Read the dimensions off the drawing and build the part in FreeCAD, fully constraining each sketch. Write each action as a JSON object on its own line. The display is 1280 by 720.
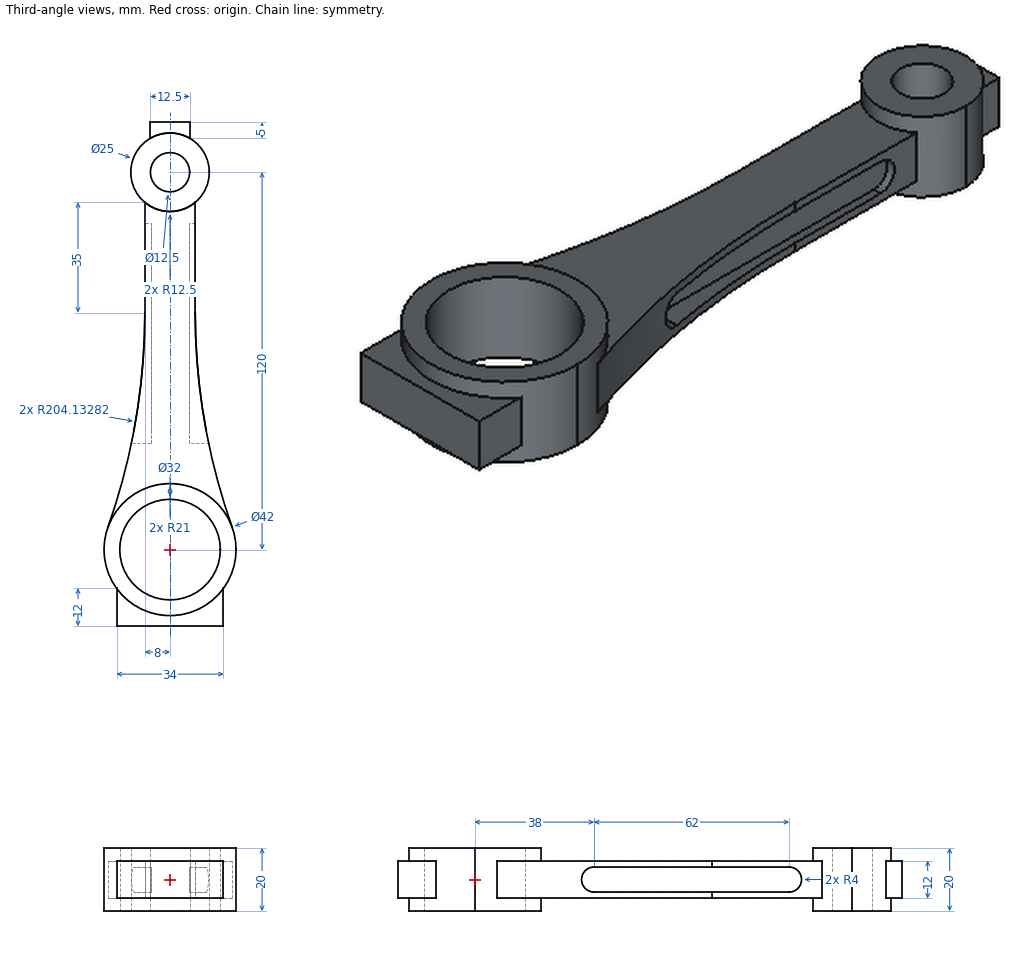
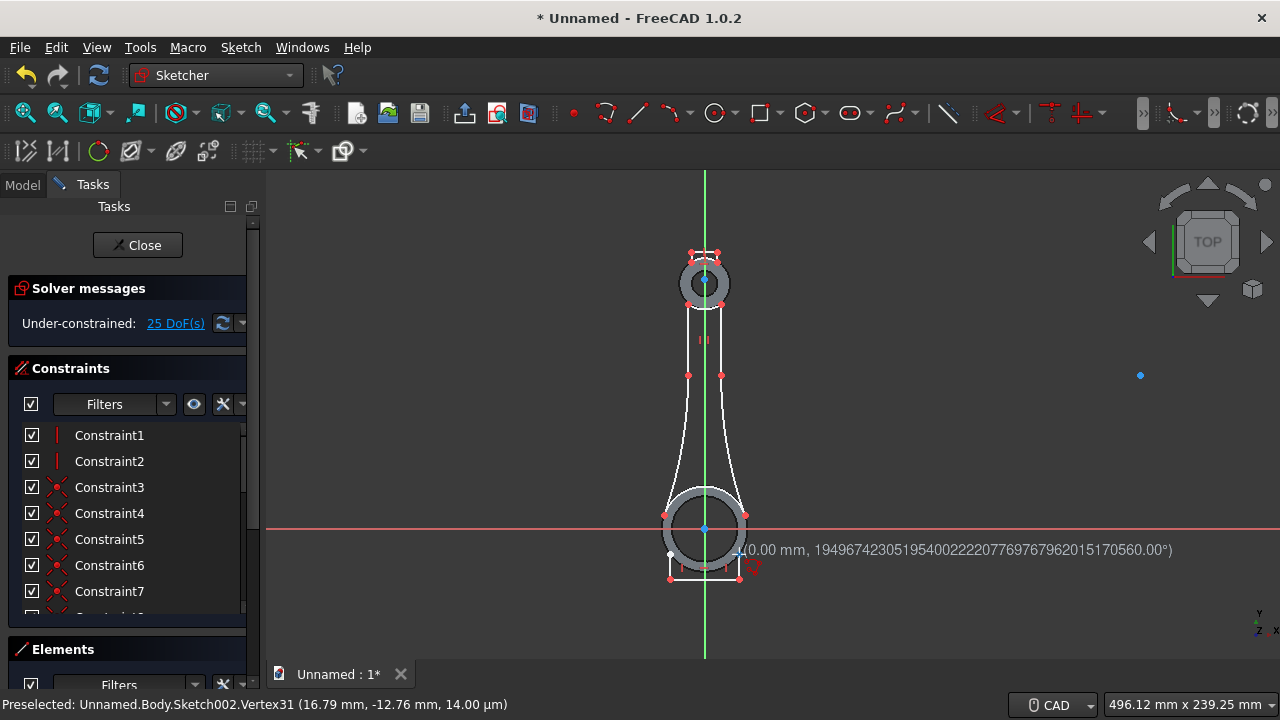
{"action": "key", "text": "g 3 a"}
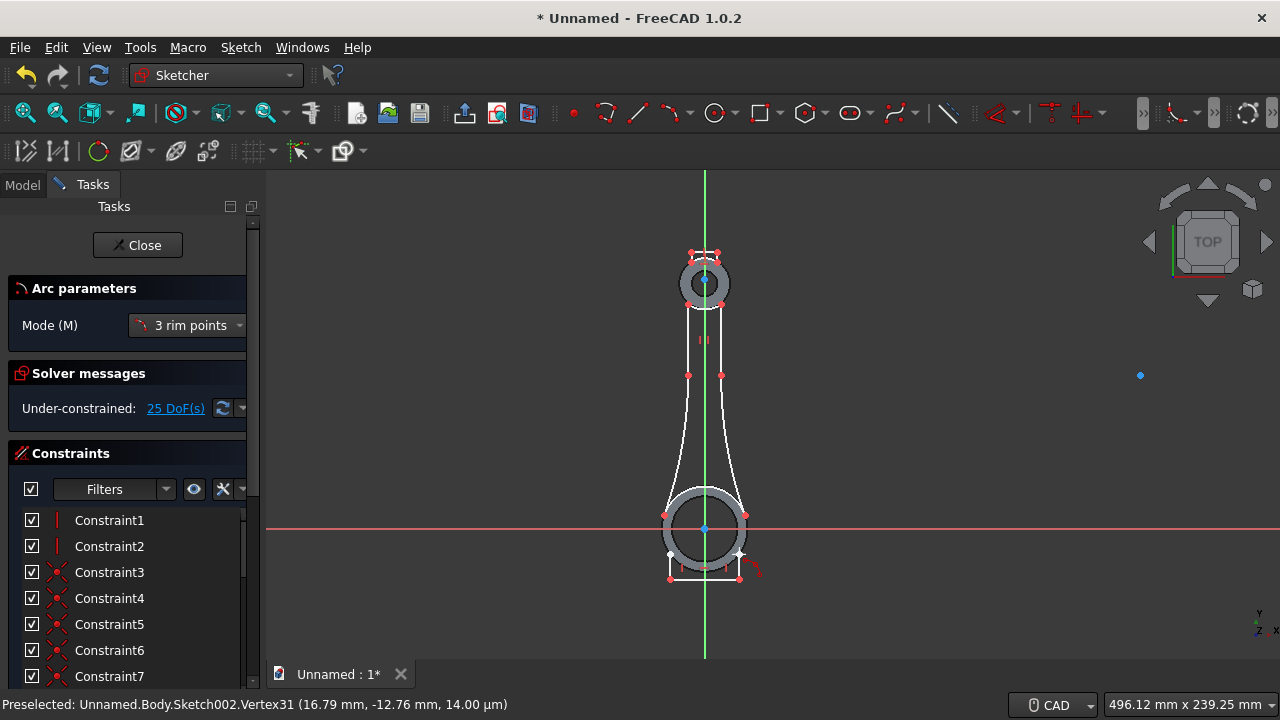
{"action": "scroll", "coordinate": [739, 554], "scroll_direction": "up", "scroll_amount": 2}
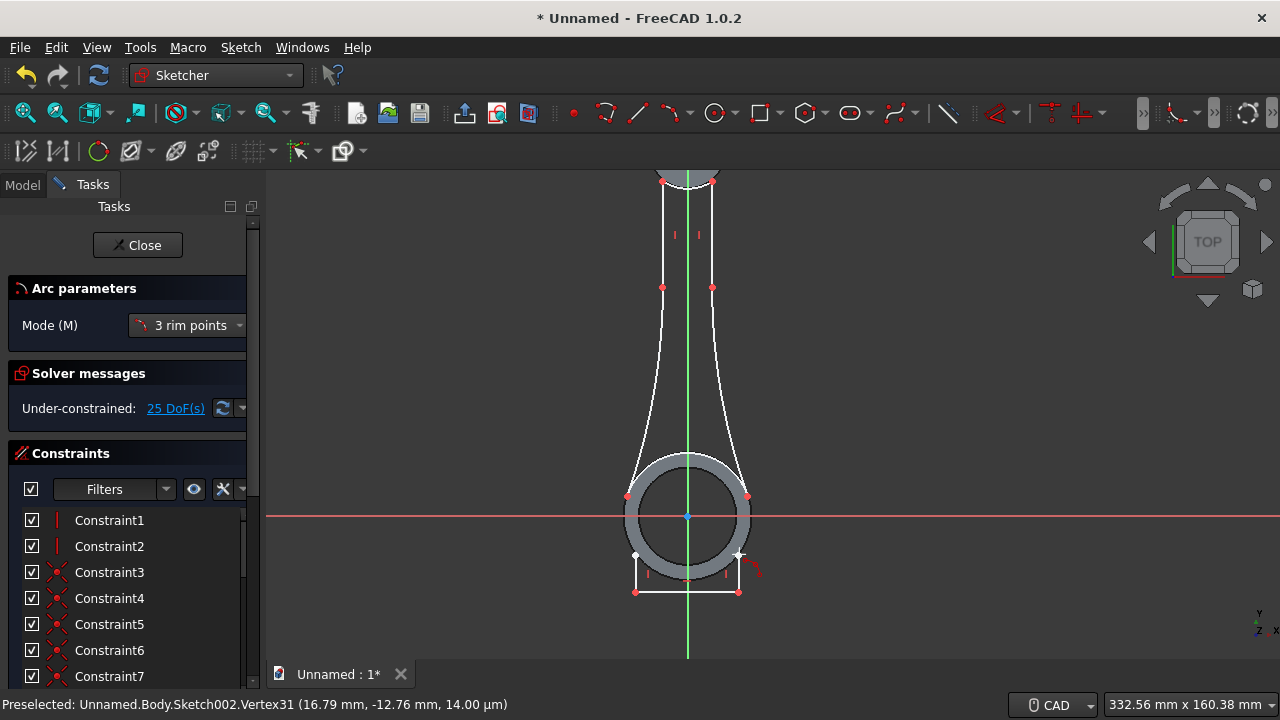
{"action": "left_click", "coordinate": [739, 555]}
{"action": "left_click", "coordinate": [636, 555]}
{"action": "left_click", "coordinate": [664, 576]}
{"action": "key", "text": "Escape"}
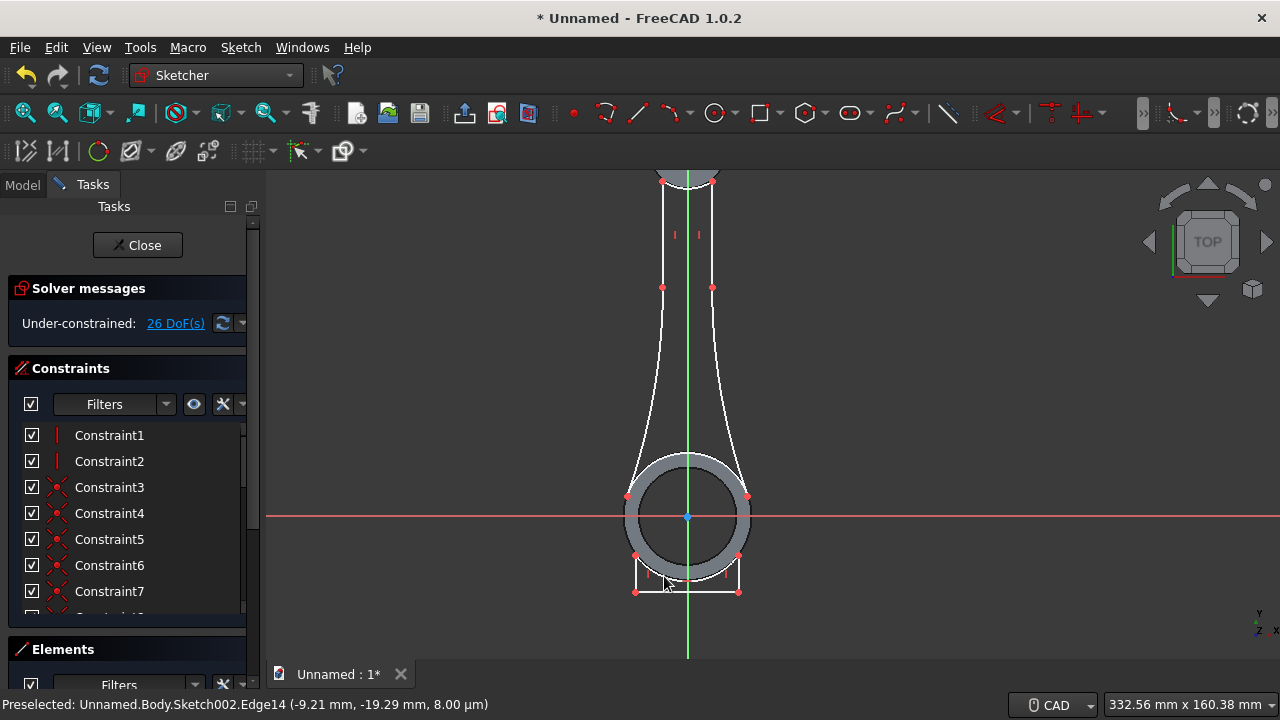
{"action": "left_click", "coordinate": [645, 435]}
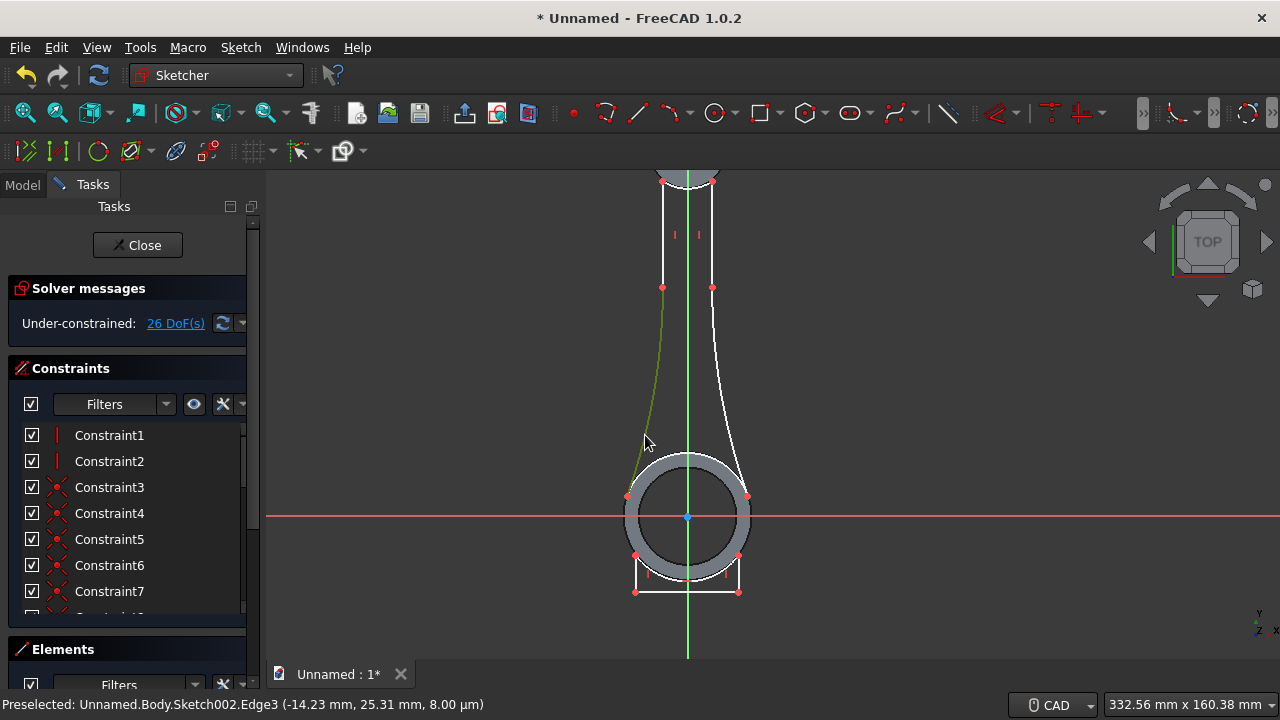
{"action": "left_click", "coordinate": [718, 461]}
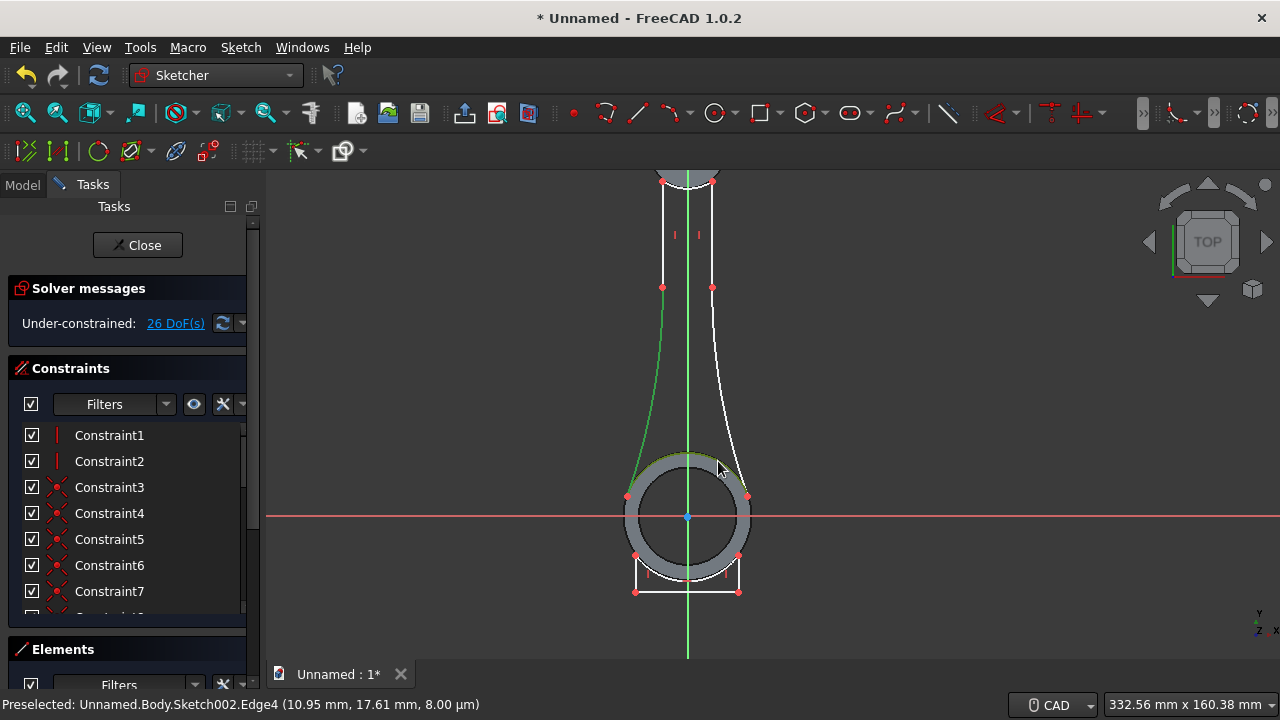
{"action": "key", "text": "t"}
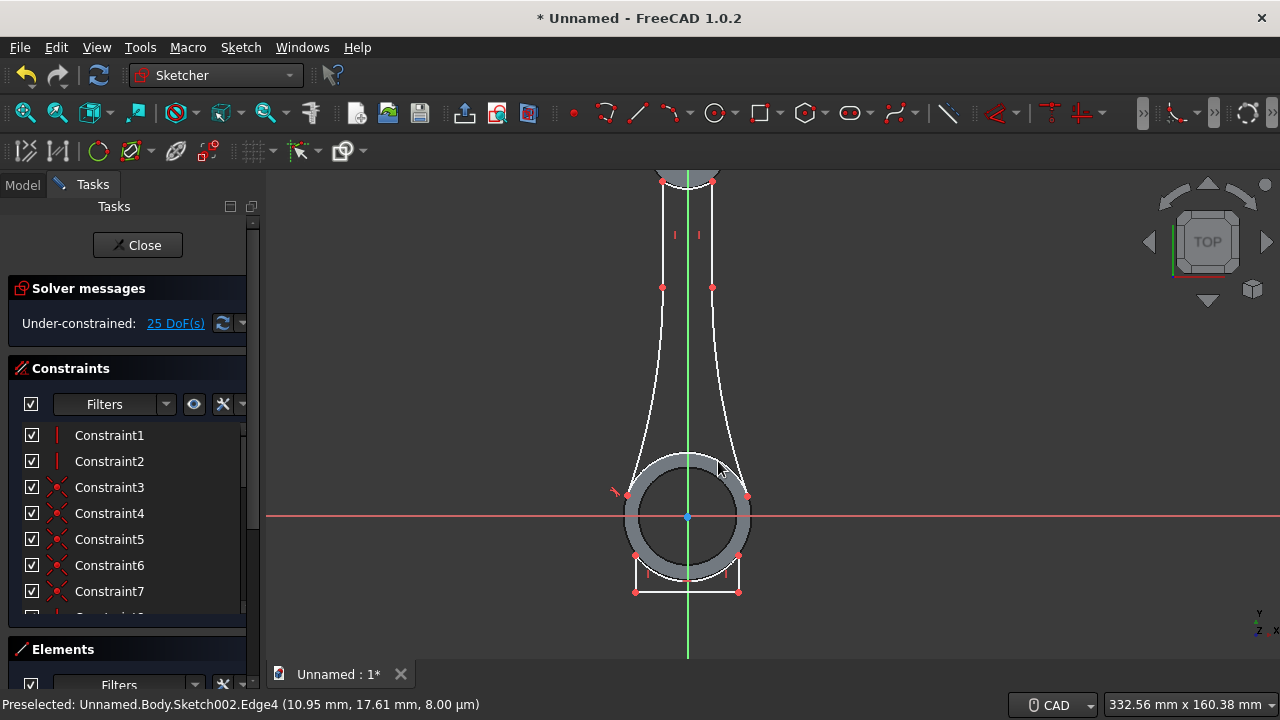
{"action": "left_click", "coordinate": [718, 461]}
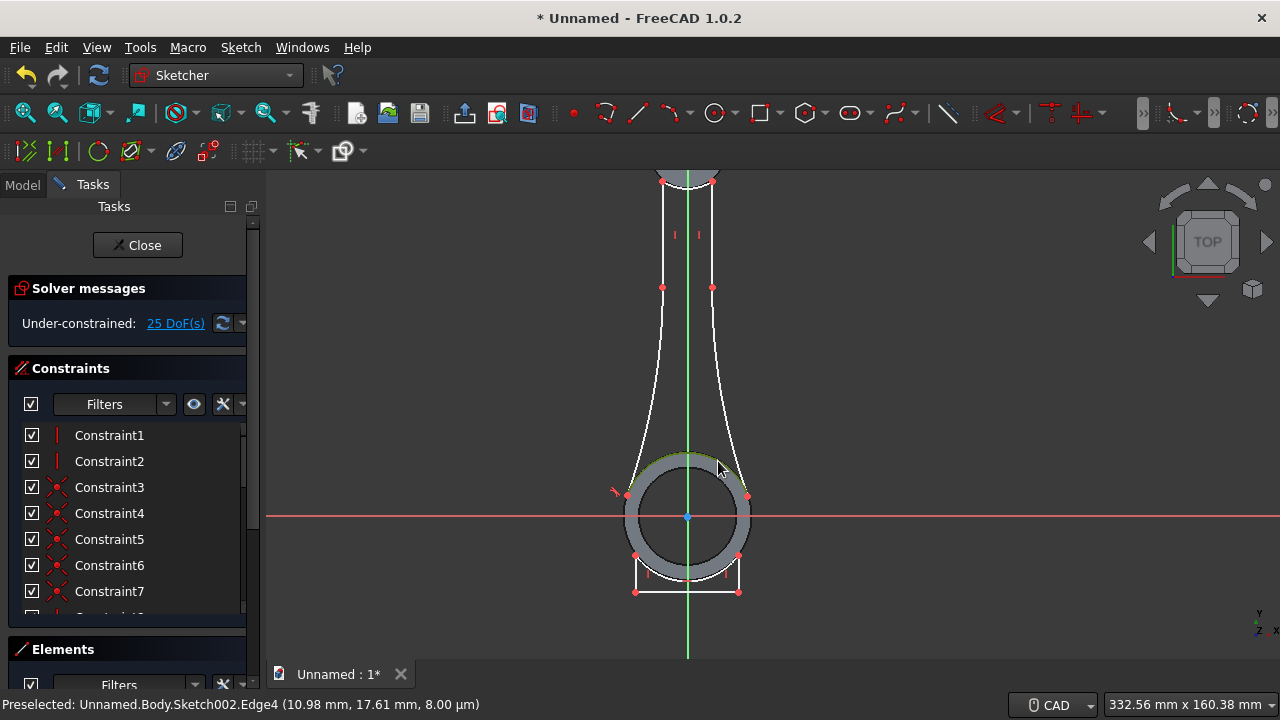
{"action": "left_click", "coordinate": [715, 351]}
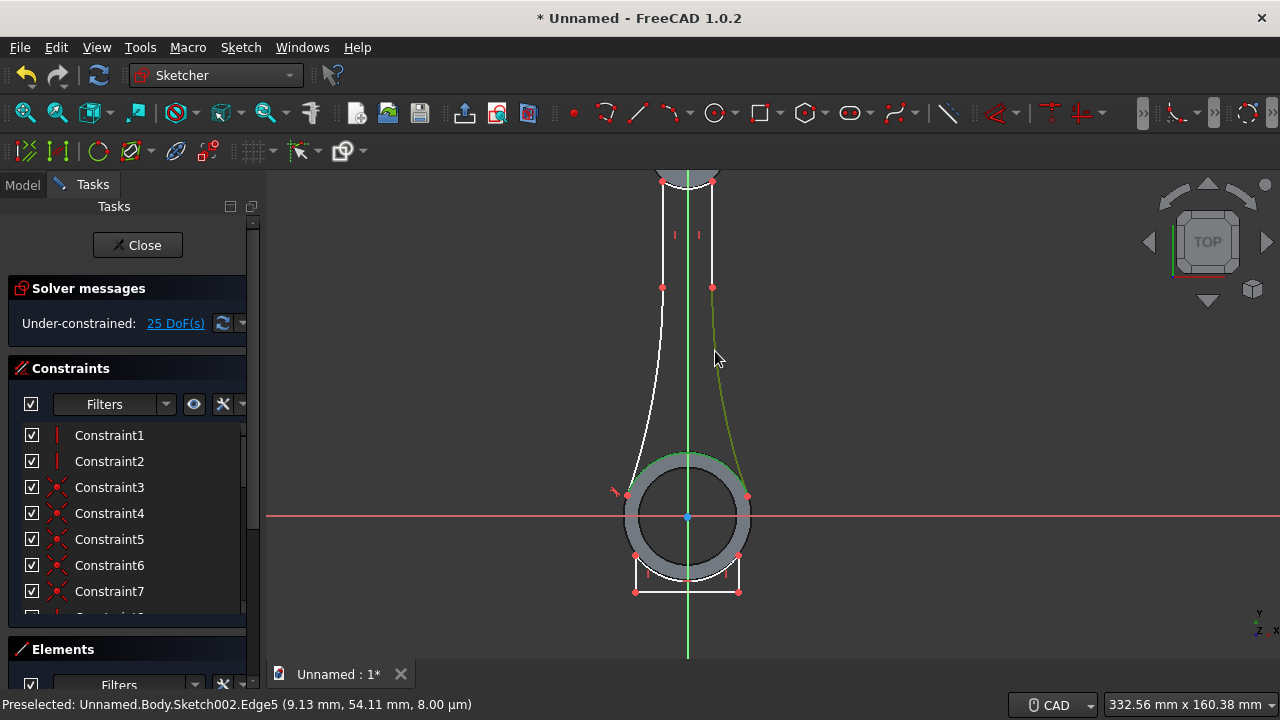
{"action": "key", "text": "t"}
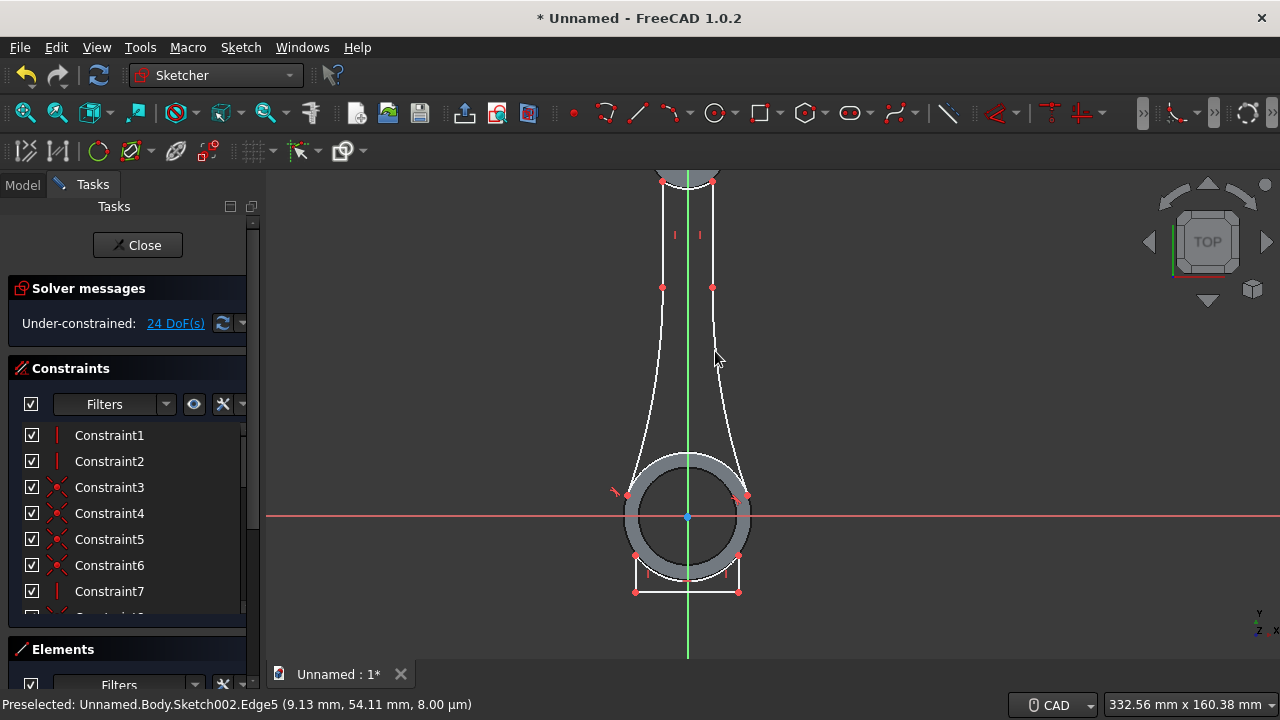
{"action": "scroll", "coordinate": [739, 553], "scroll_direction": "down", "scroll_amount": 2}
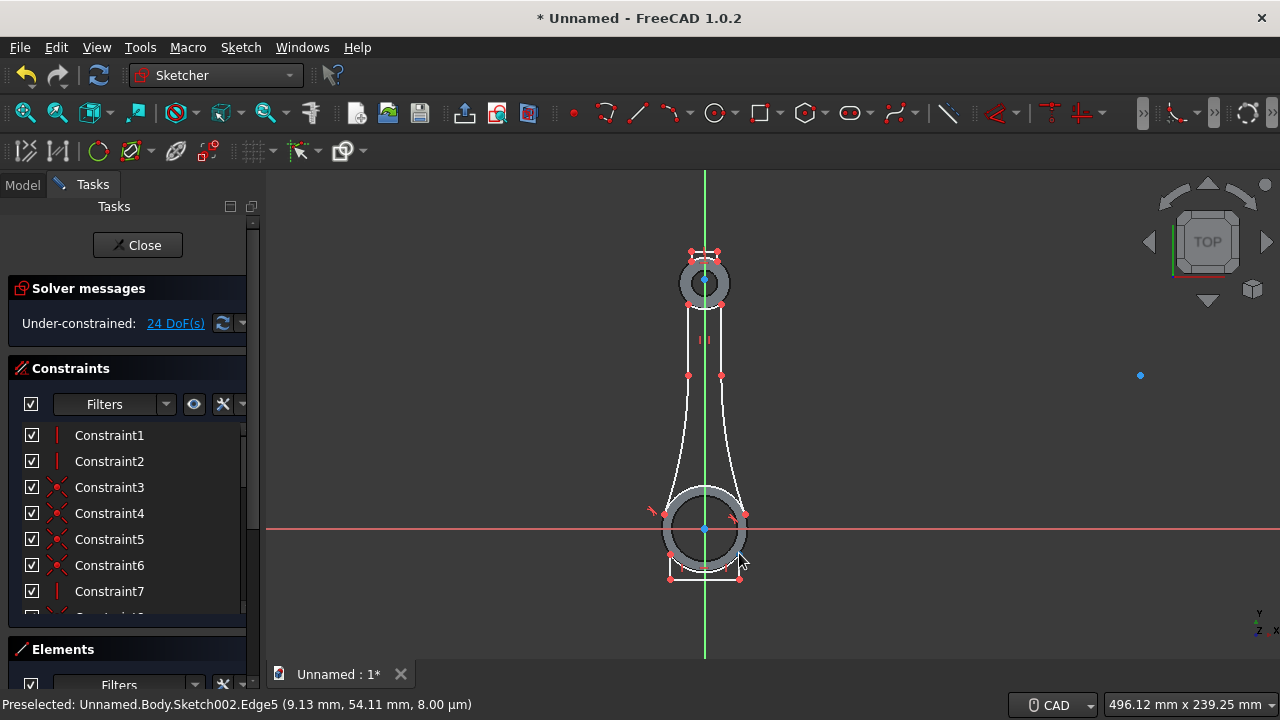
{"action": "scroll", "coordinate": [698, 308], "scroll_direction": "up", "scroll_amount": 4}